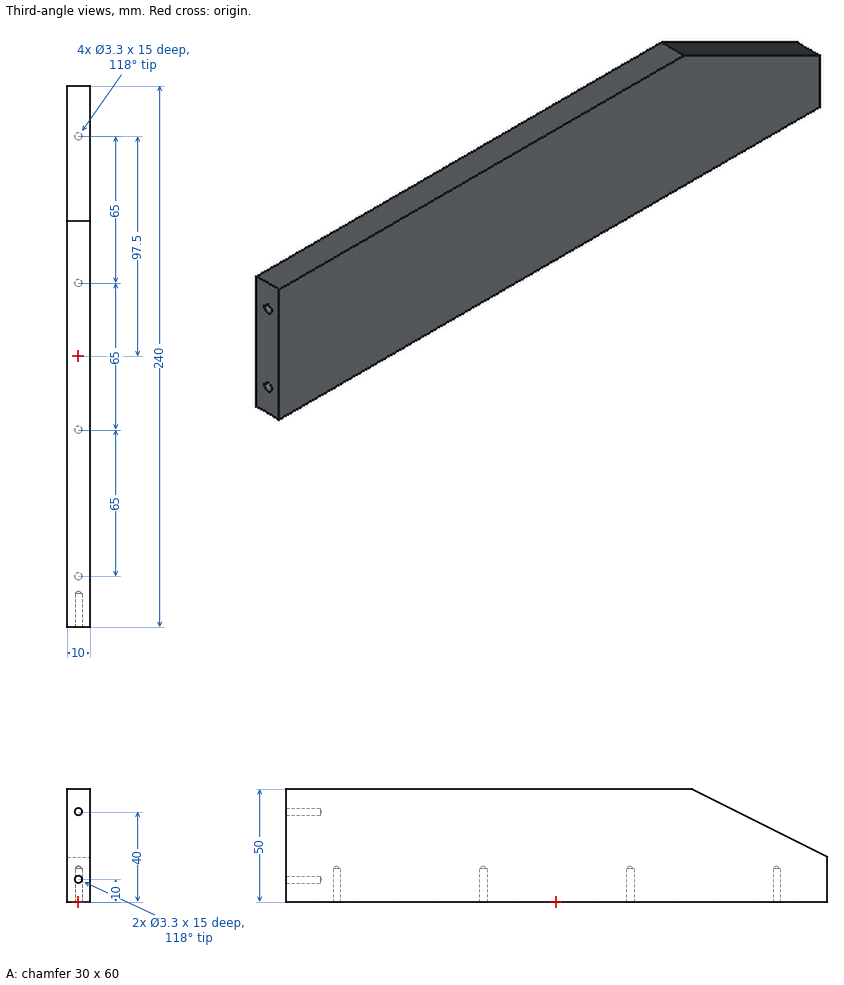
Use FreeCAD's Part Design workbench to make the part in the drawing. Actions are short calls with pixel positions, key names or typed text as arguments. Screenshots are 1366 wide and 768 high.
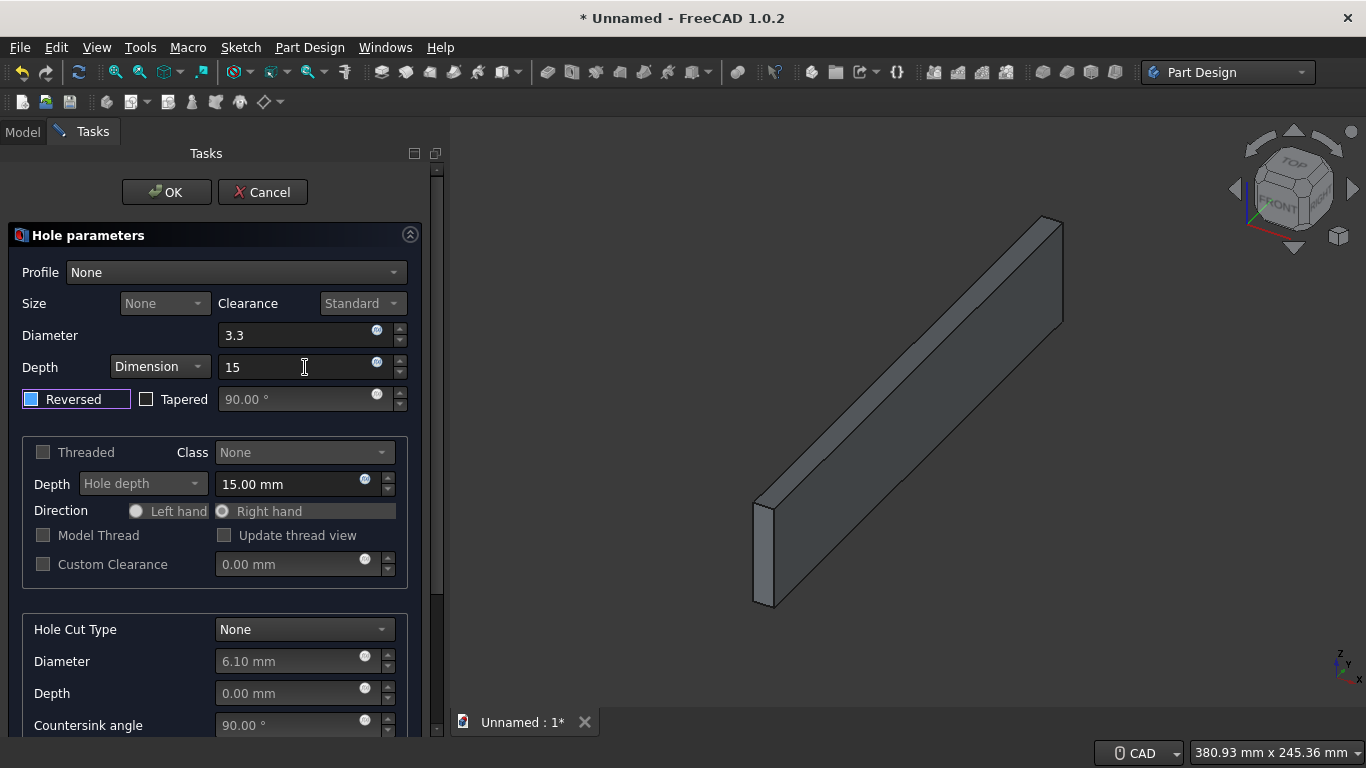
click(30, 399)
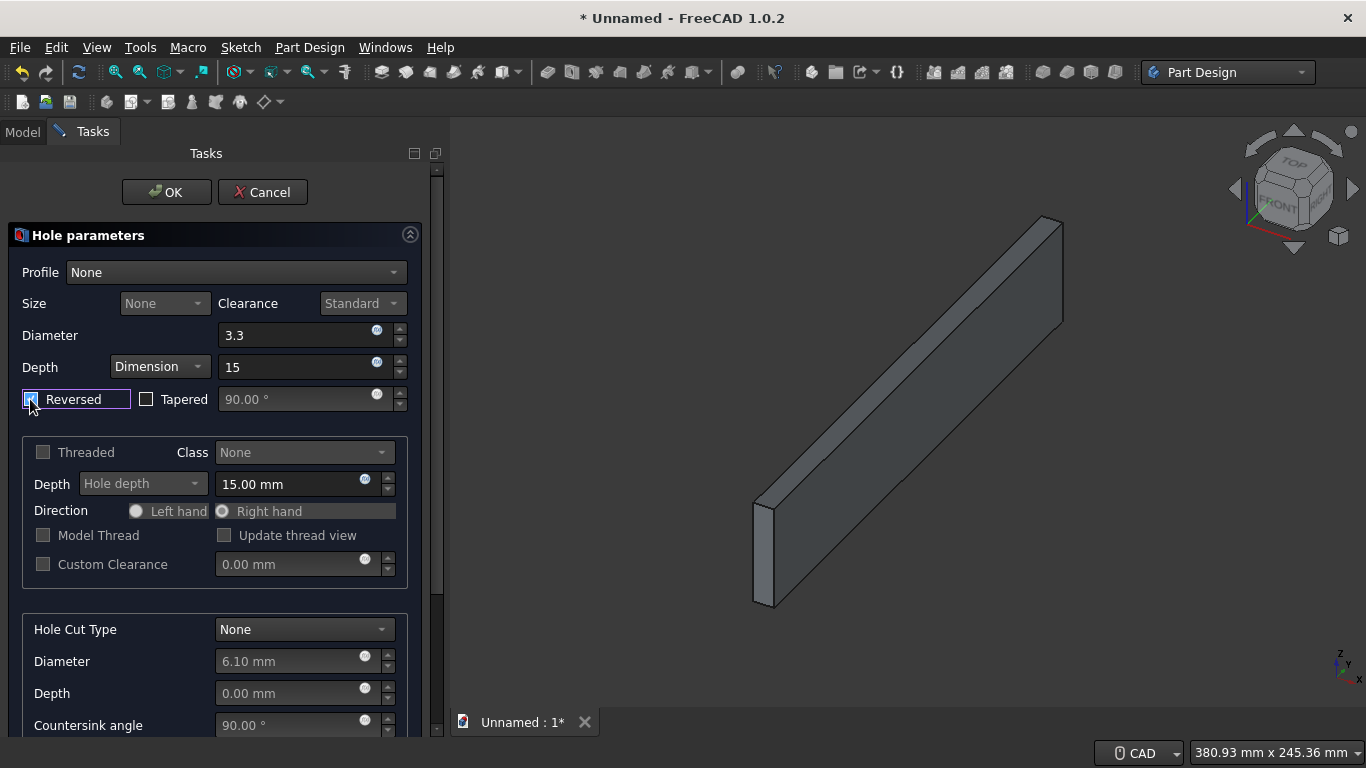
click(167, 192)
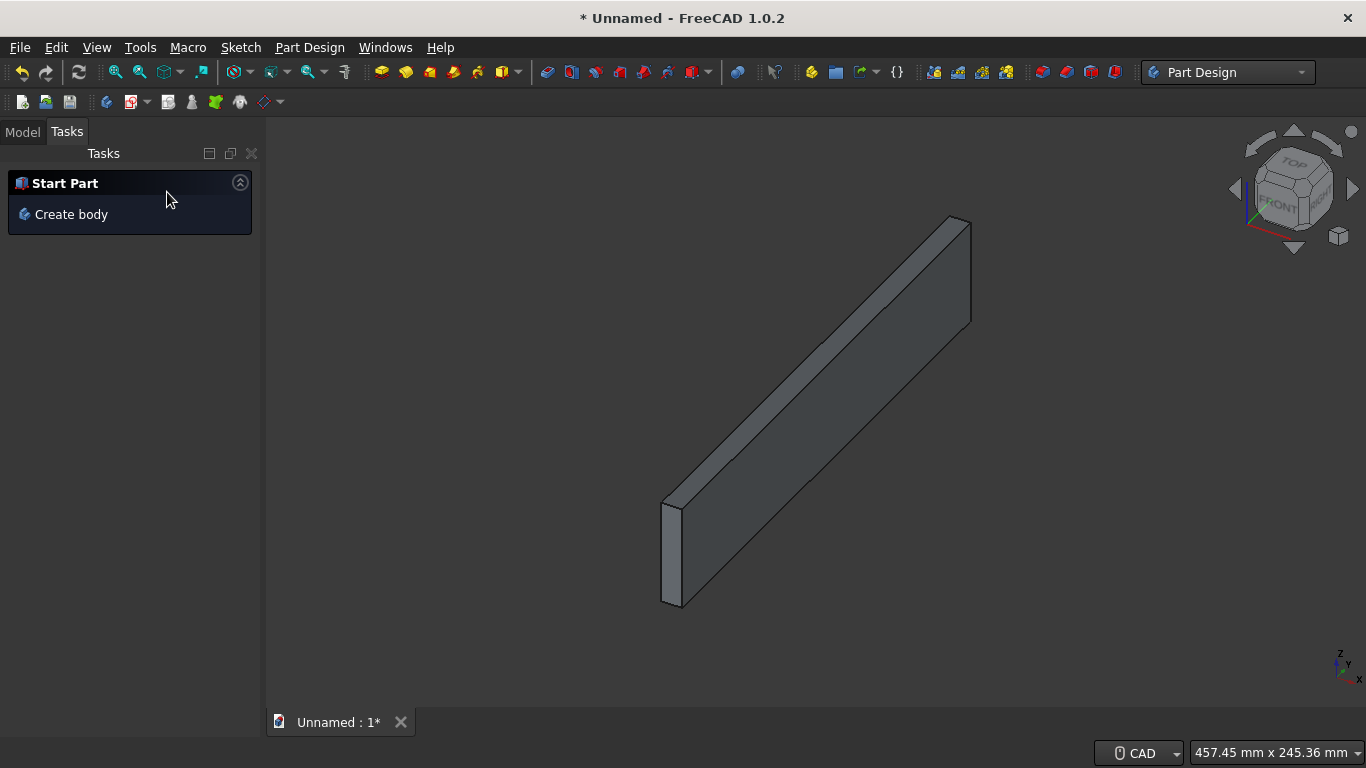
click(672, 526)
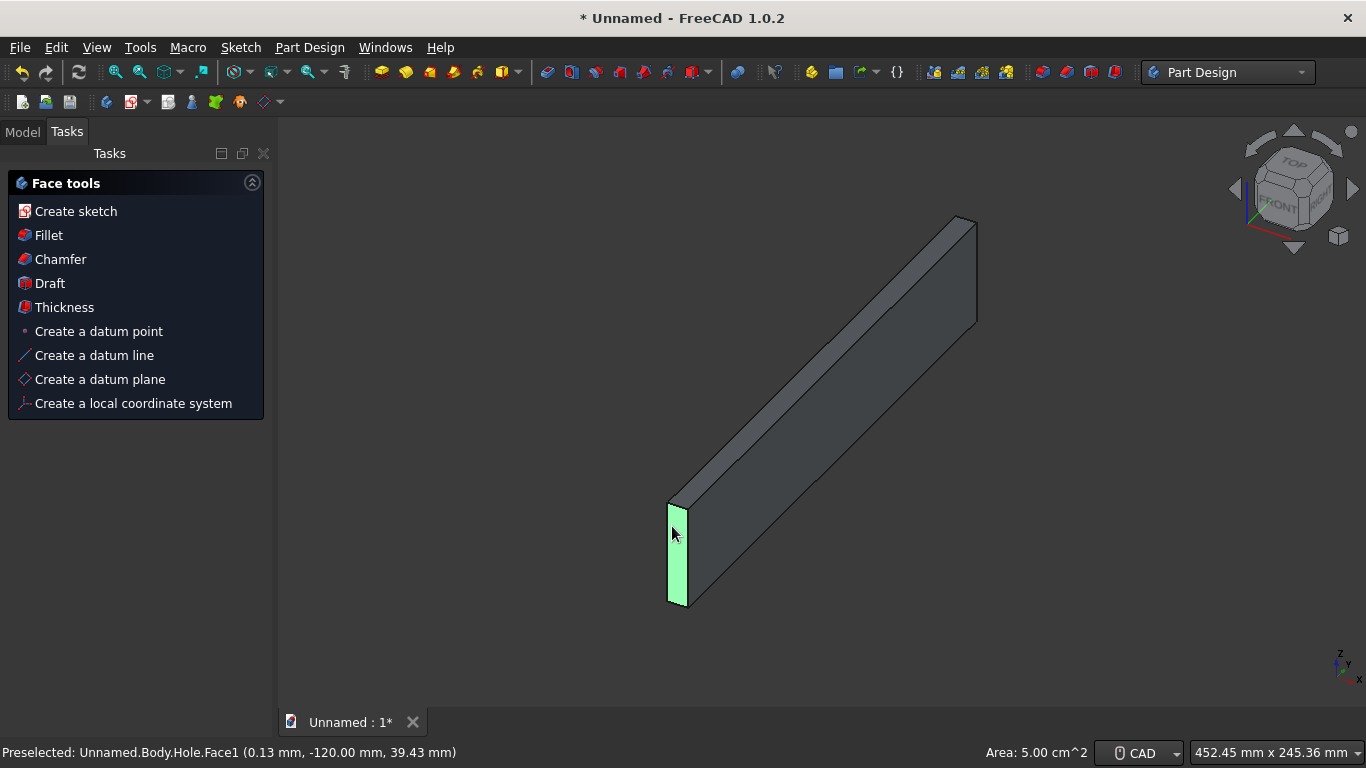
click(132, 102)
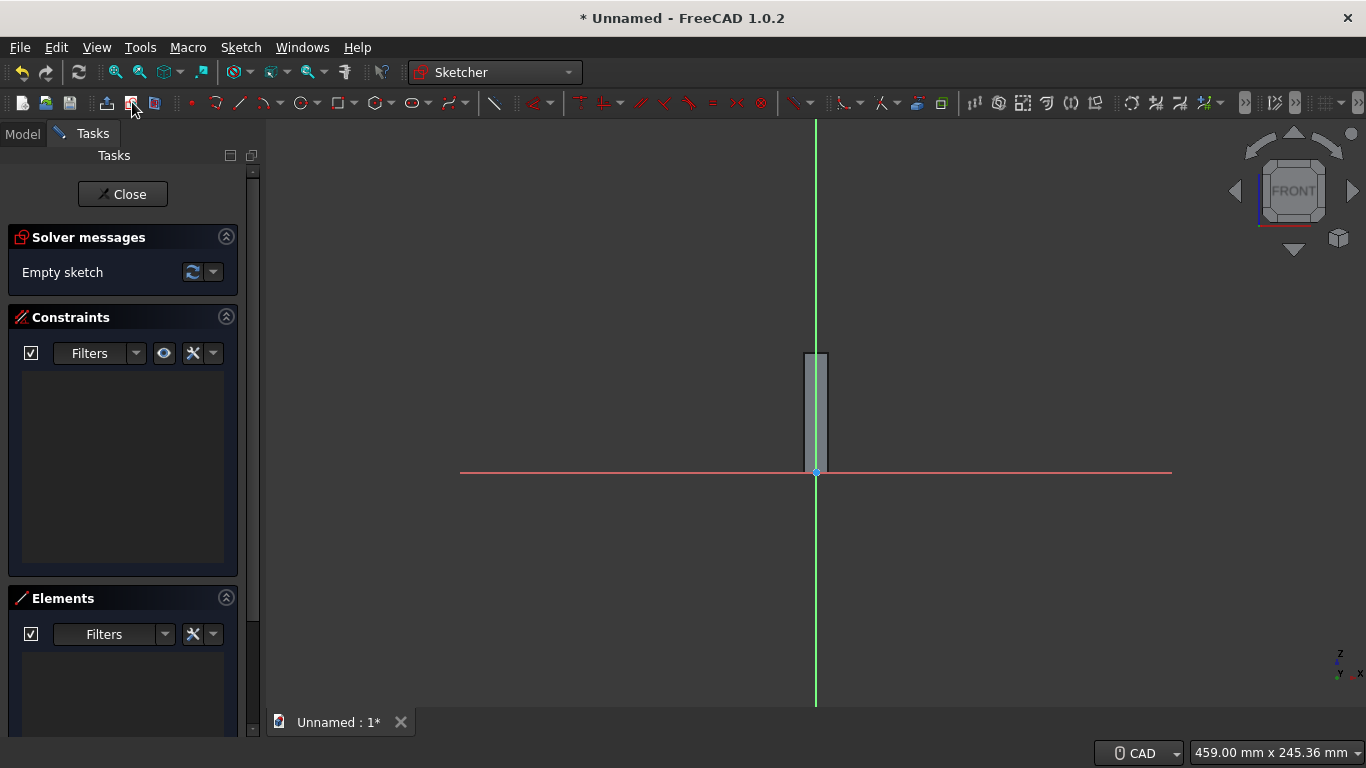
scroll(838, 426, up, 7)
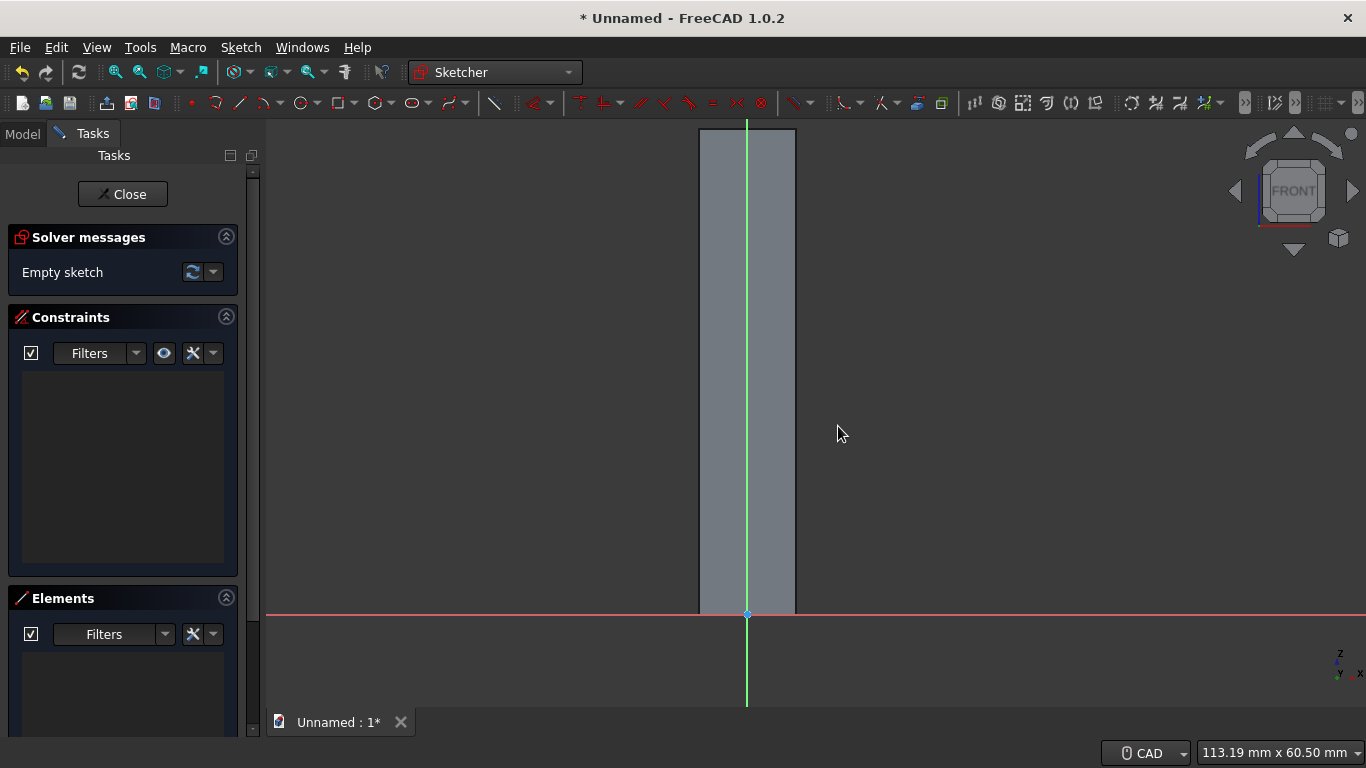
click(302, 104)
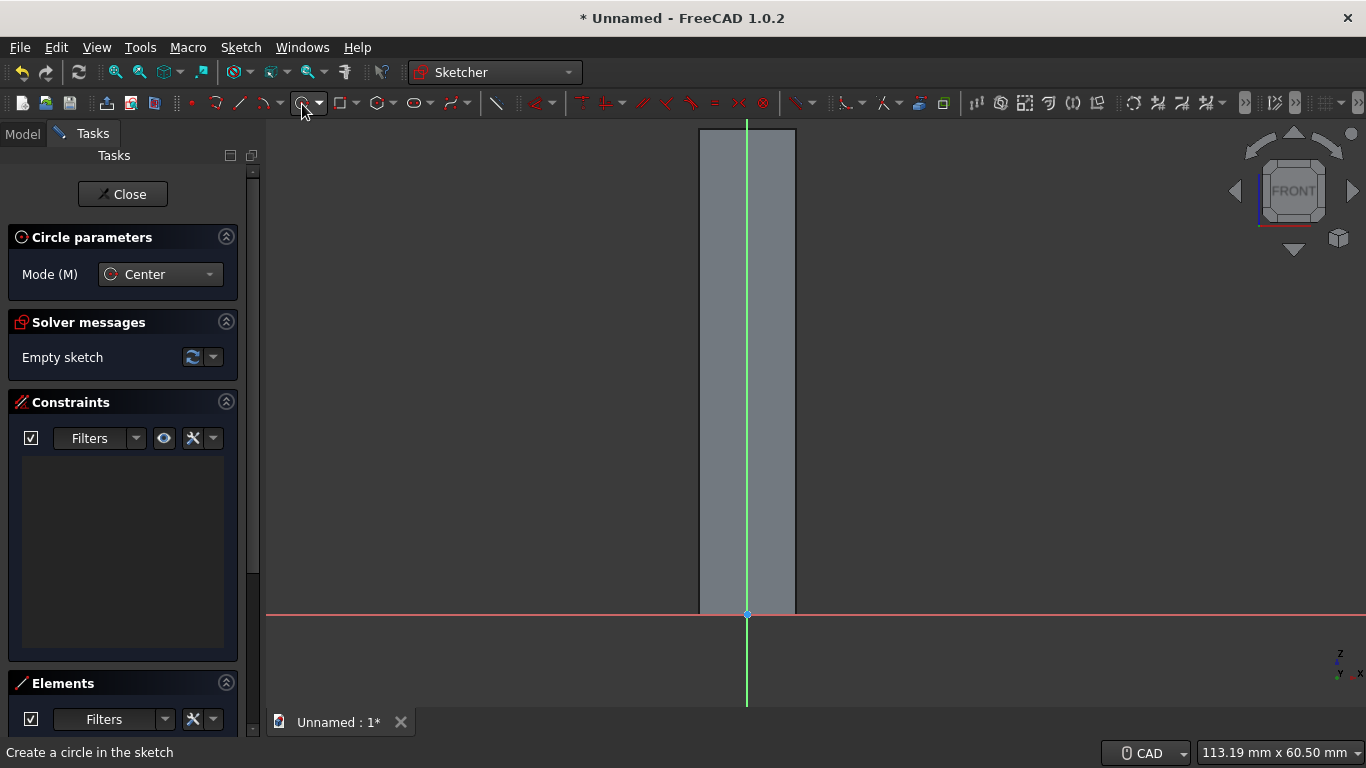
scroll(747, 517, up, 2)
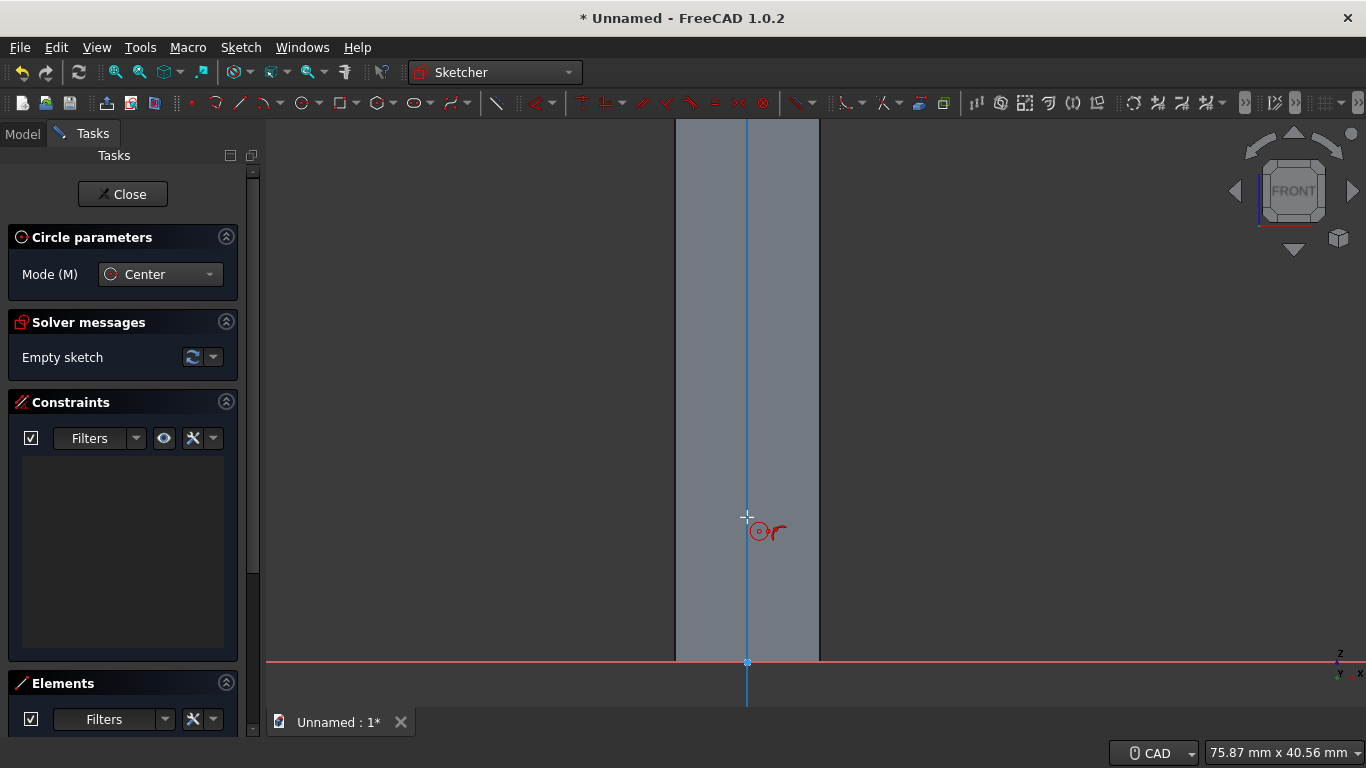
click(747, 517)
move(764, 500)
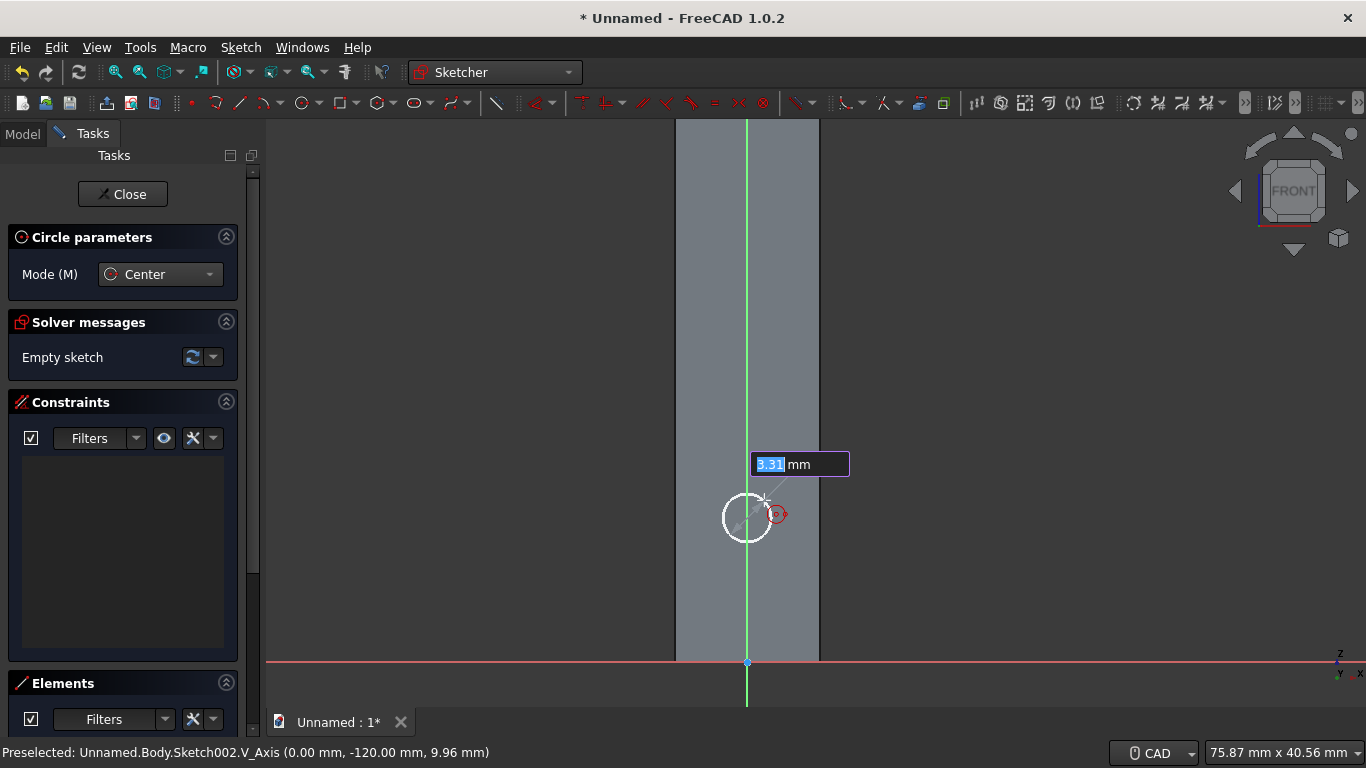
text(3.3)
key(Return)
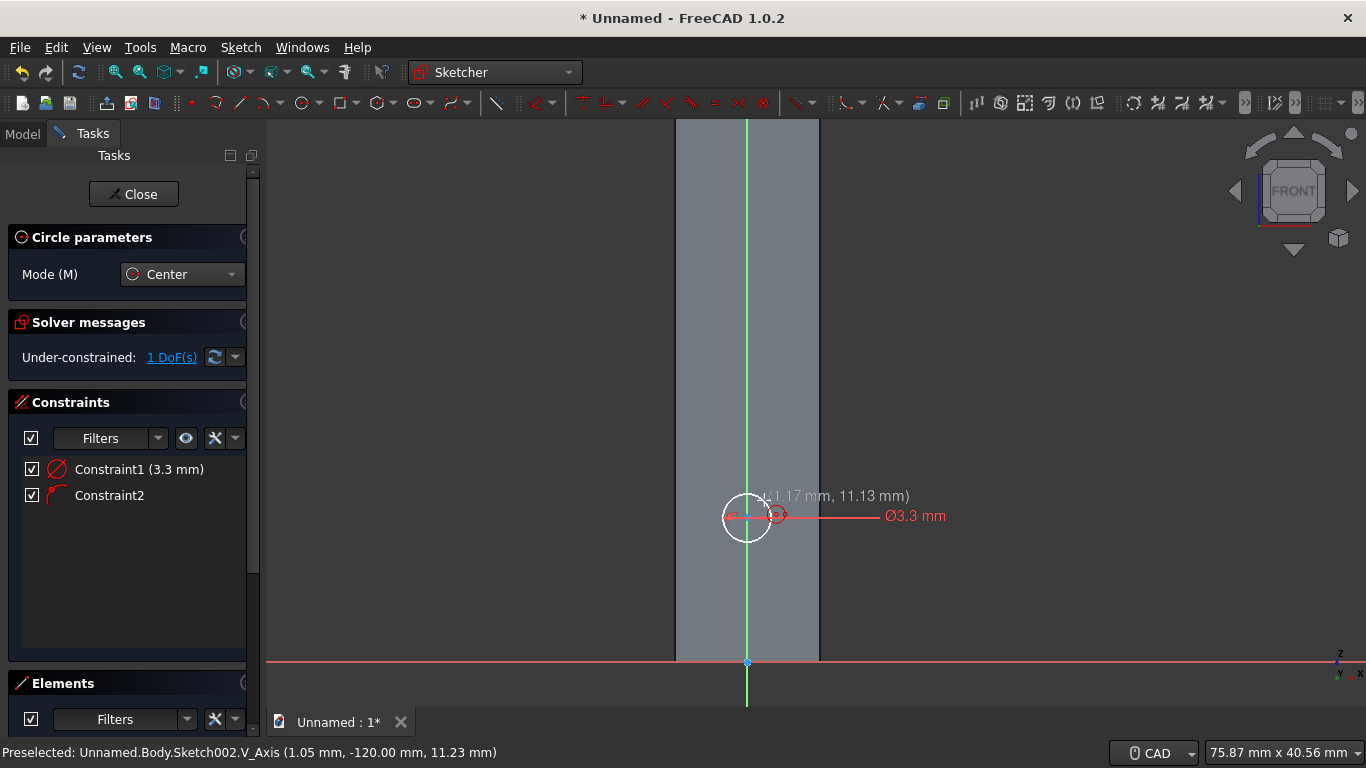
scroll(748, 520, down, 2)